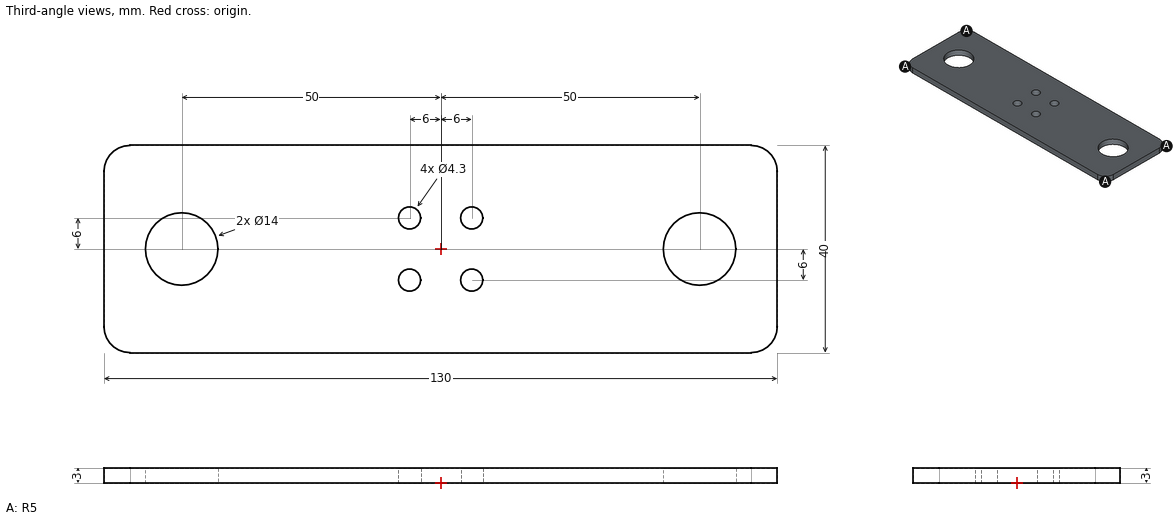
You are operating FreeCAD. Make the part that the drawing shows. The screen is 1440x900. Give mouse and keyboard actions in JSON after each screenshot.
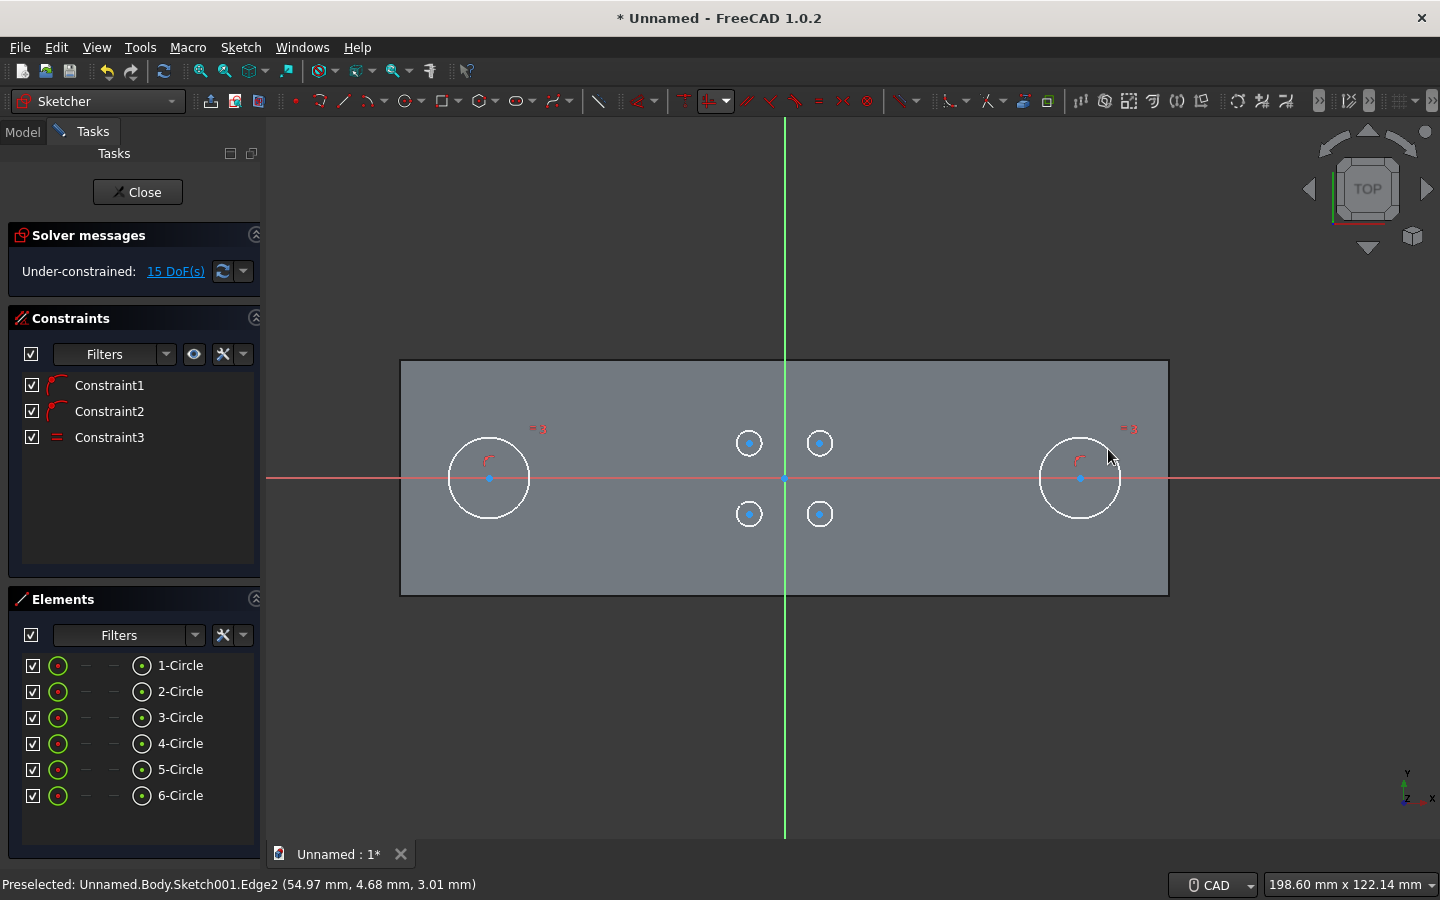
{"action": "left_click", "coordinate": [758, 434]}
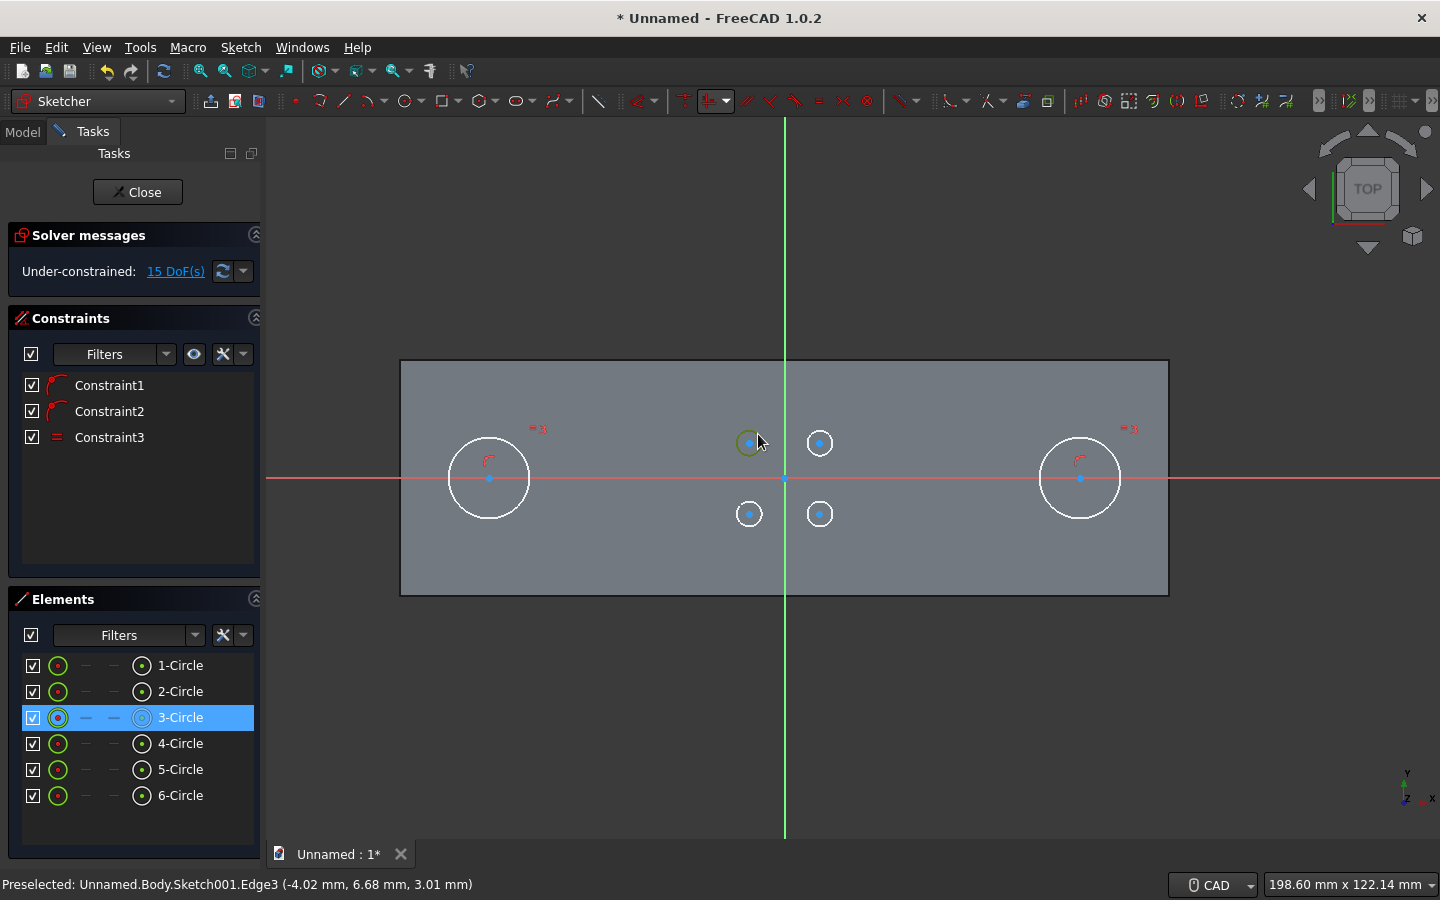
{"action": "left_click", "coordinate": [829, 434]}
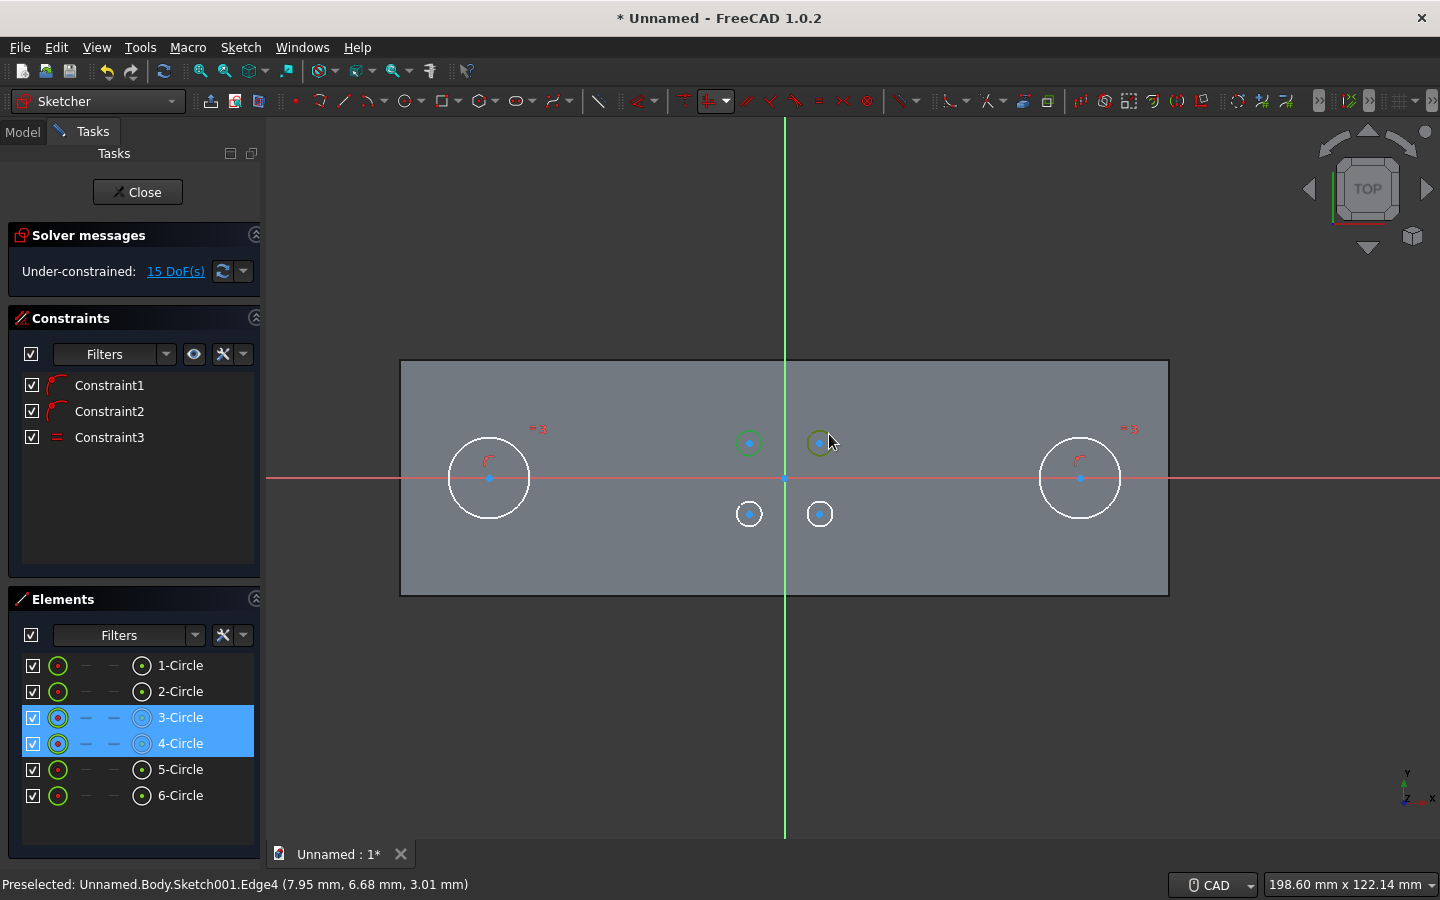
{"action": "left_click", "coordinate": [829, 505]}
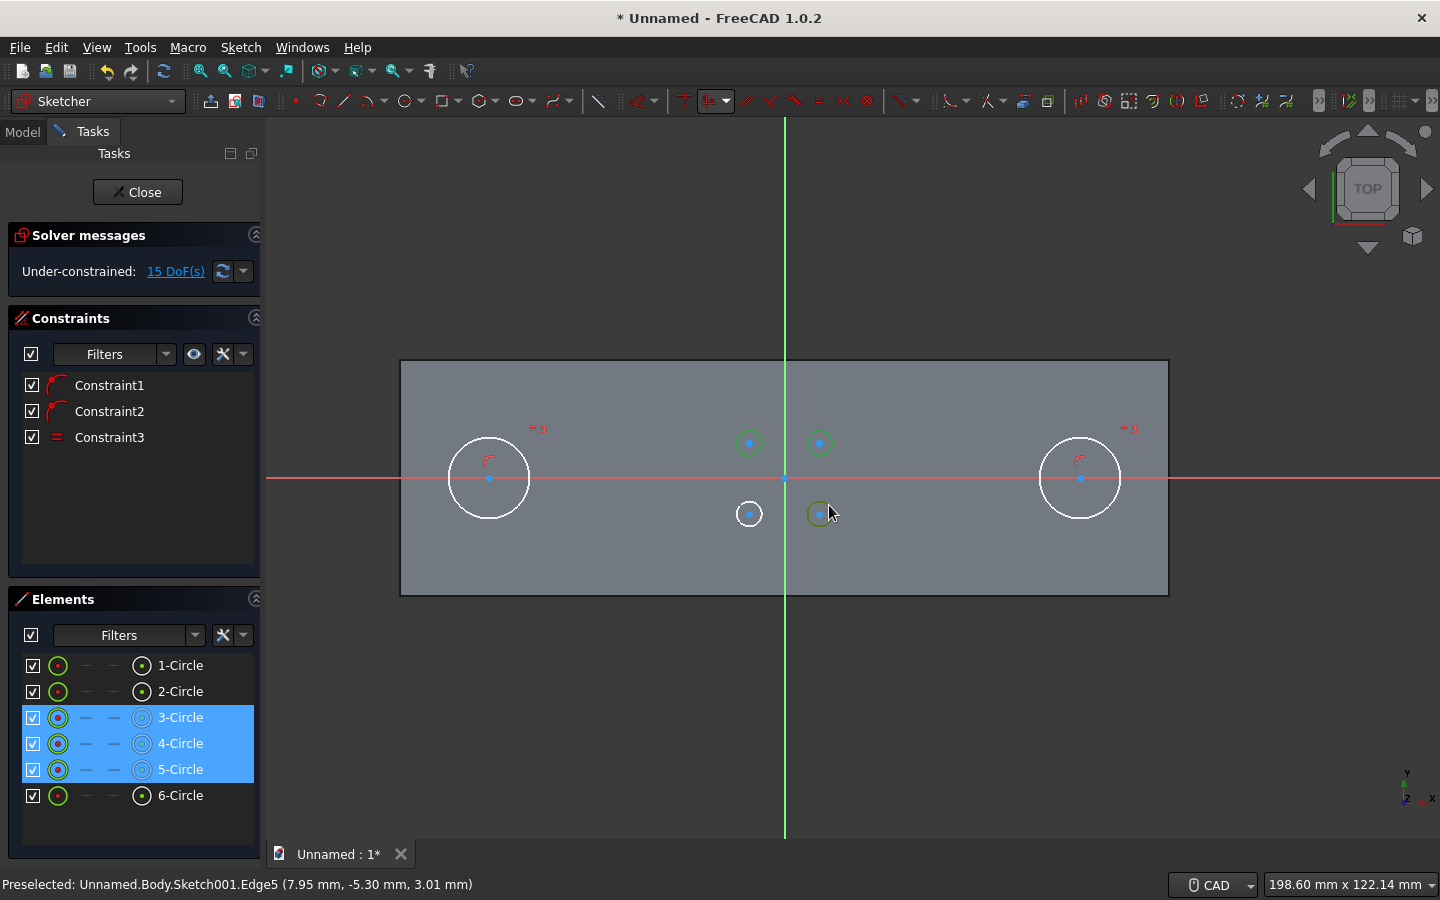
{"action": "left_click", "coordinate": [758, 505]}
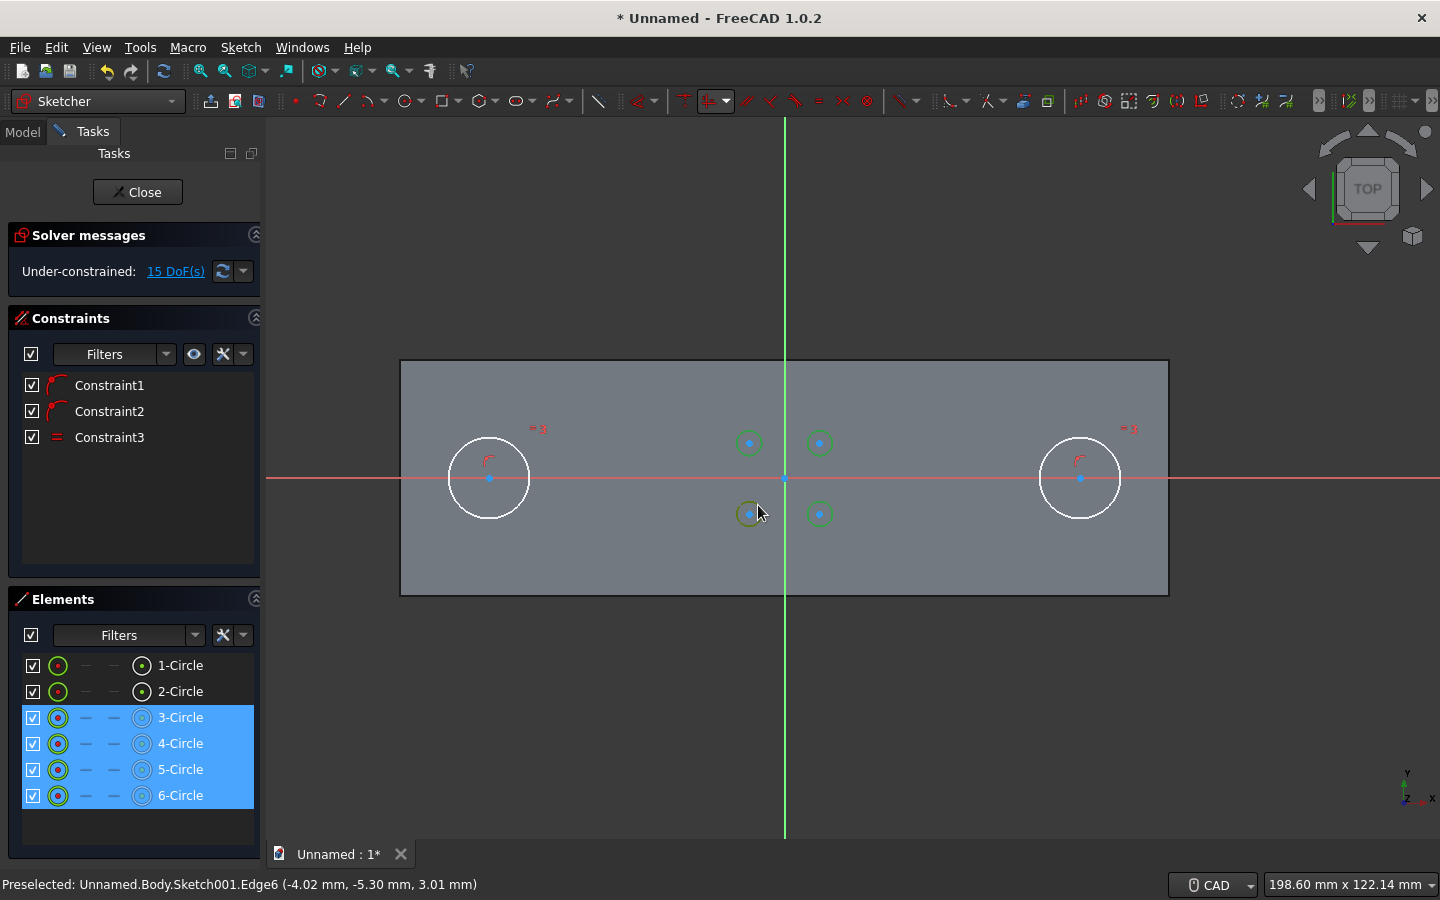
{"action": "left_click", "coordinate": [820, 102]}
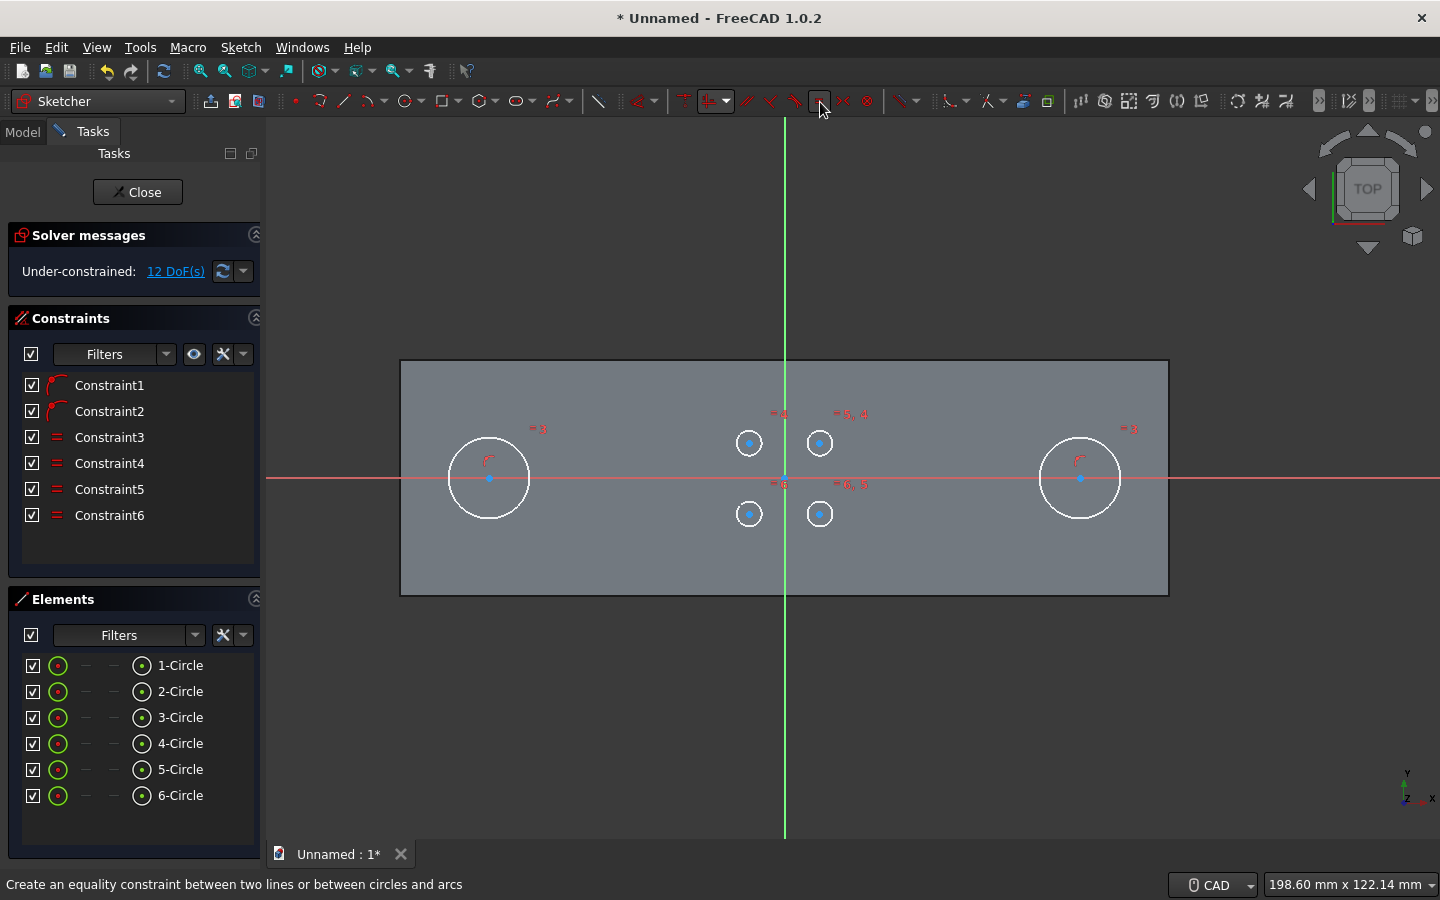
{"action": "left_click", "coordinate": [517, 449]}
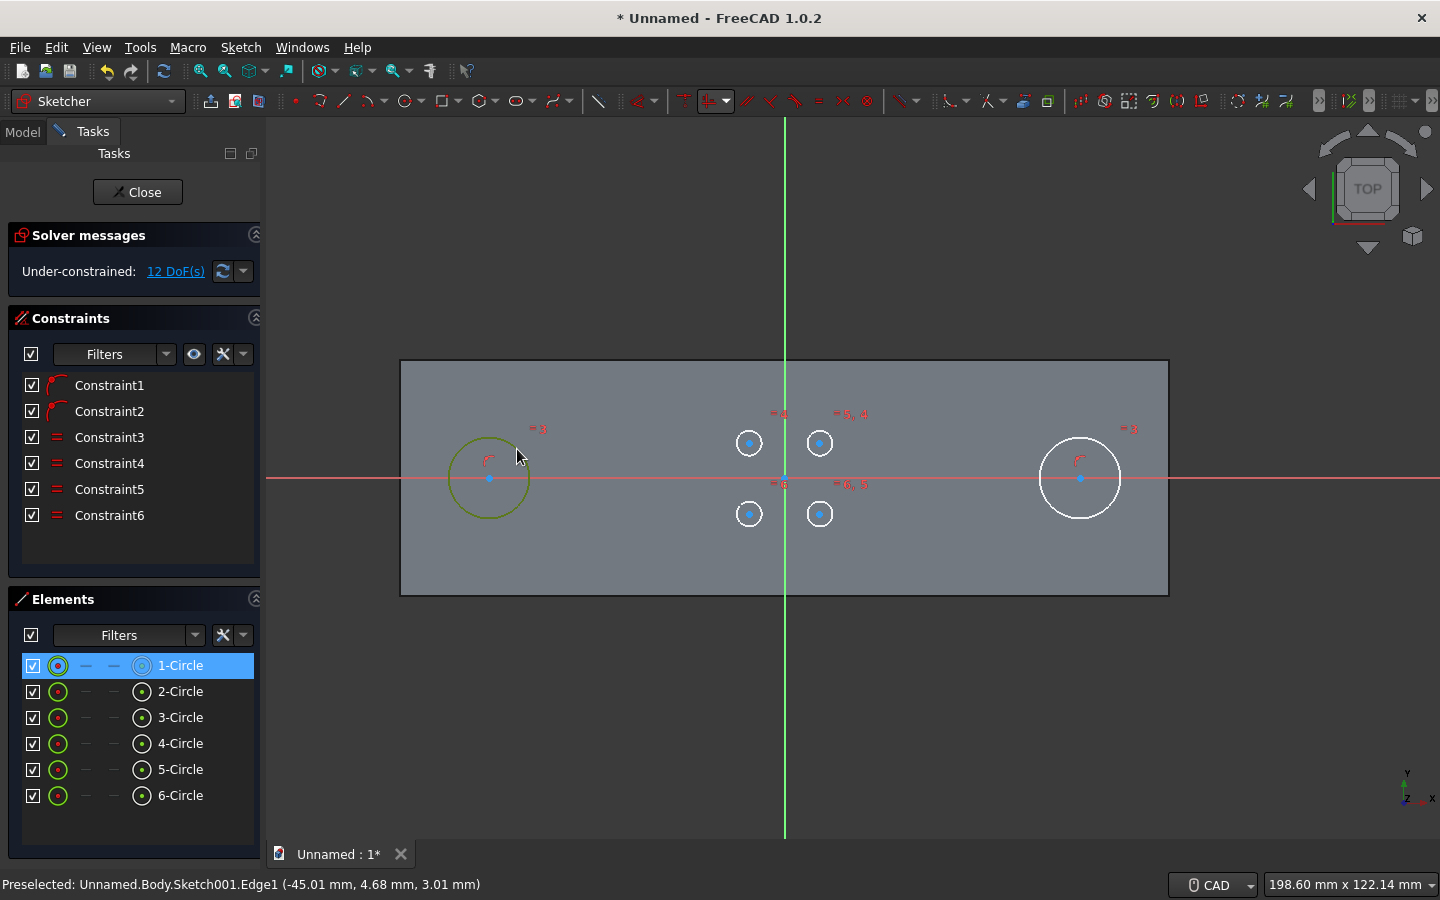
{"action": "key", "text": "k o"}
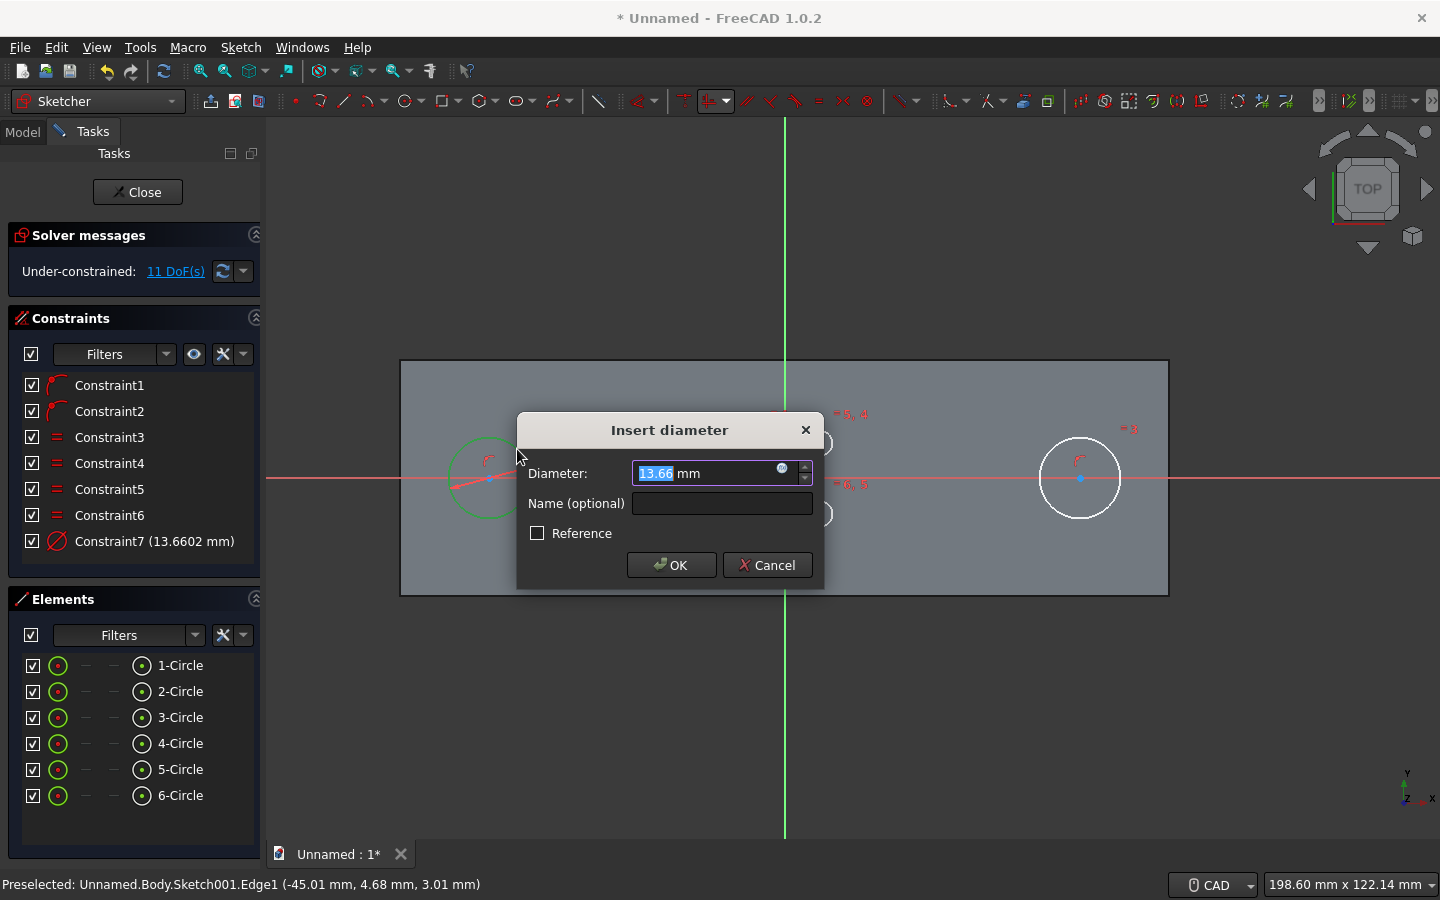
{"action": "type", "text": "14"}
{"action": "key", "text": "Return"}